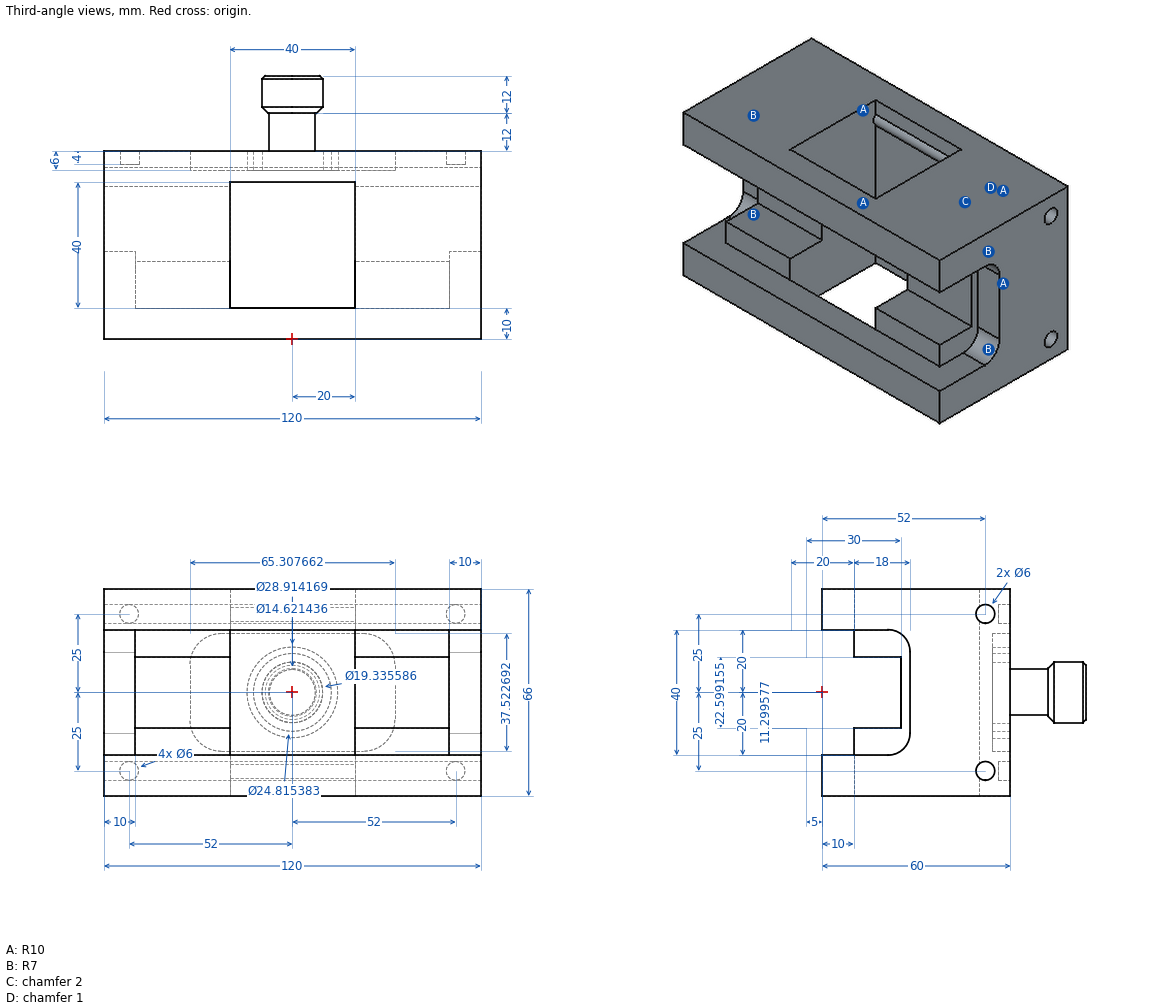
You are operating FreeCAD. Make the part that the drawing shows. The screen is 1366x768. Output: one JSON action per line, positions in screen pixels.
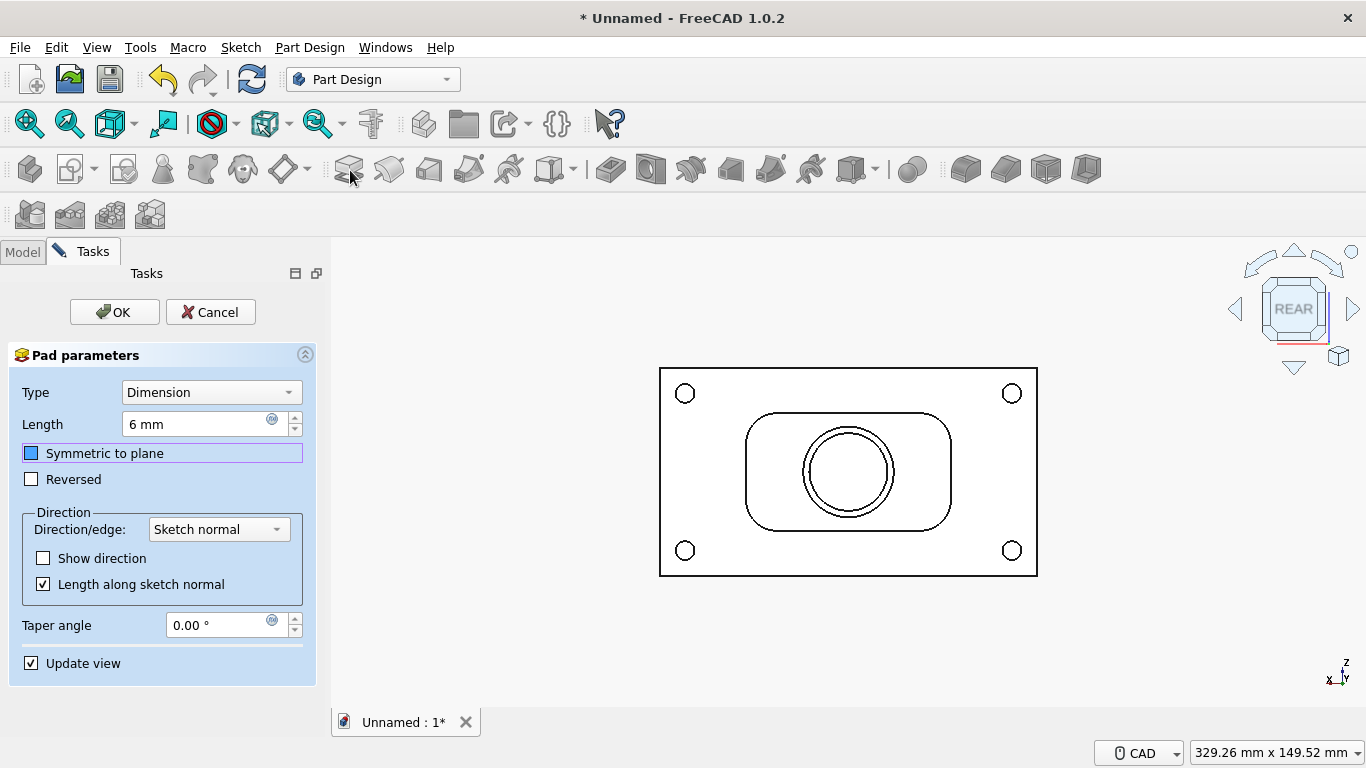
{"action": "left_click", "coordinate": [115, 312]}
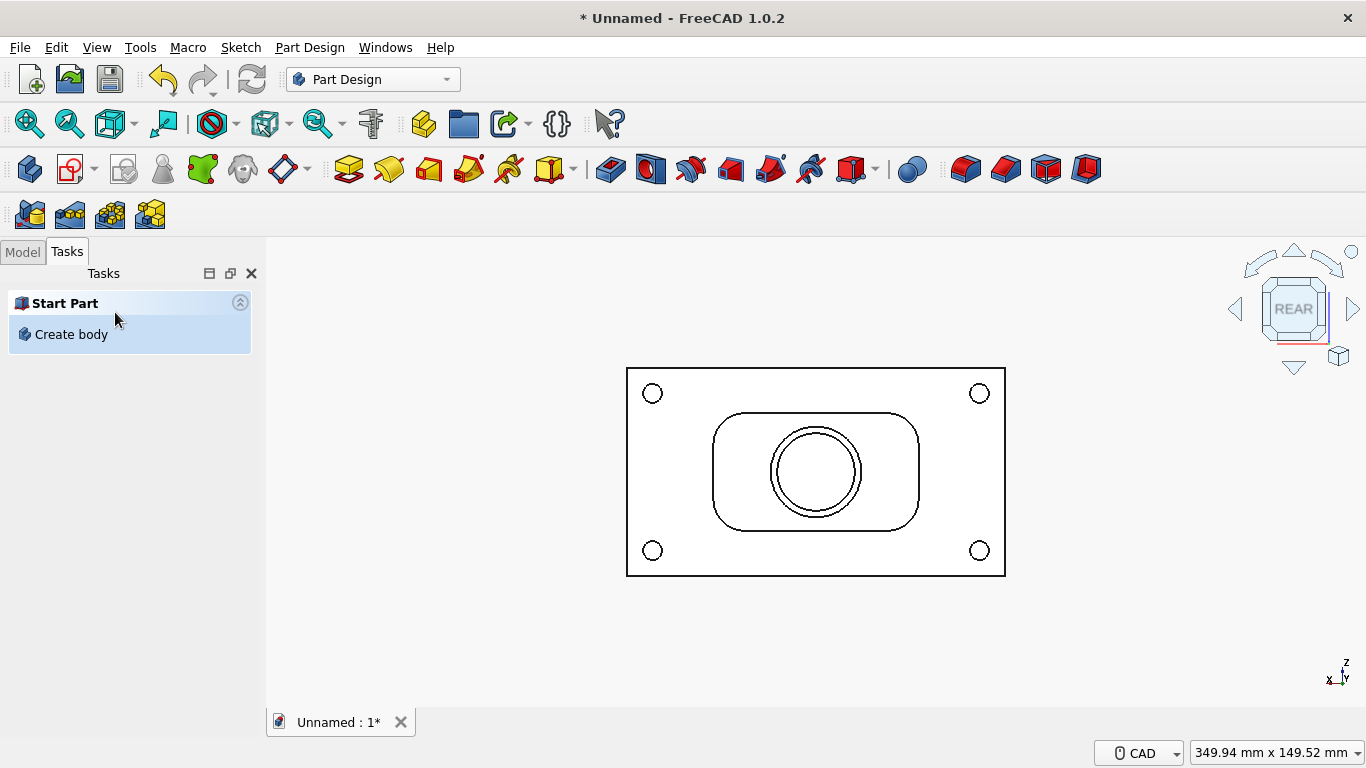
{"action": "left_click", "coordinate": [30, 124]}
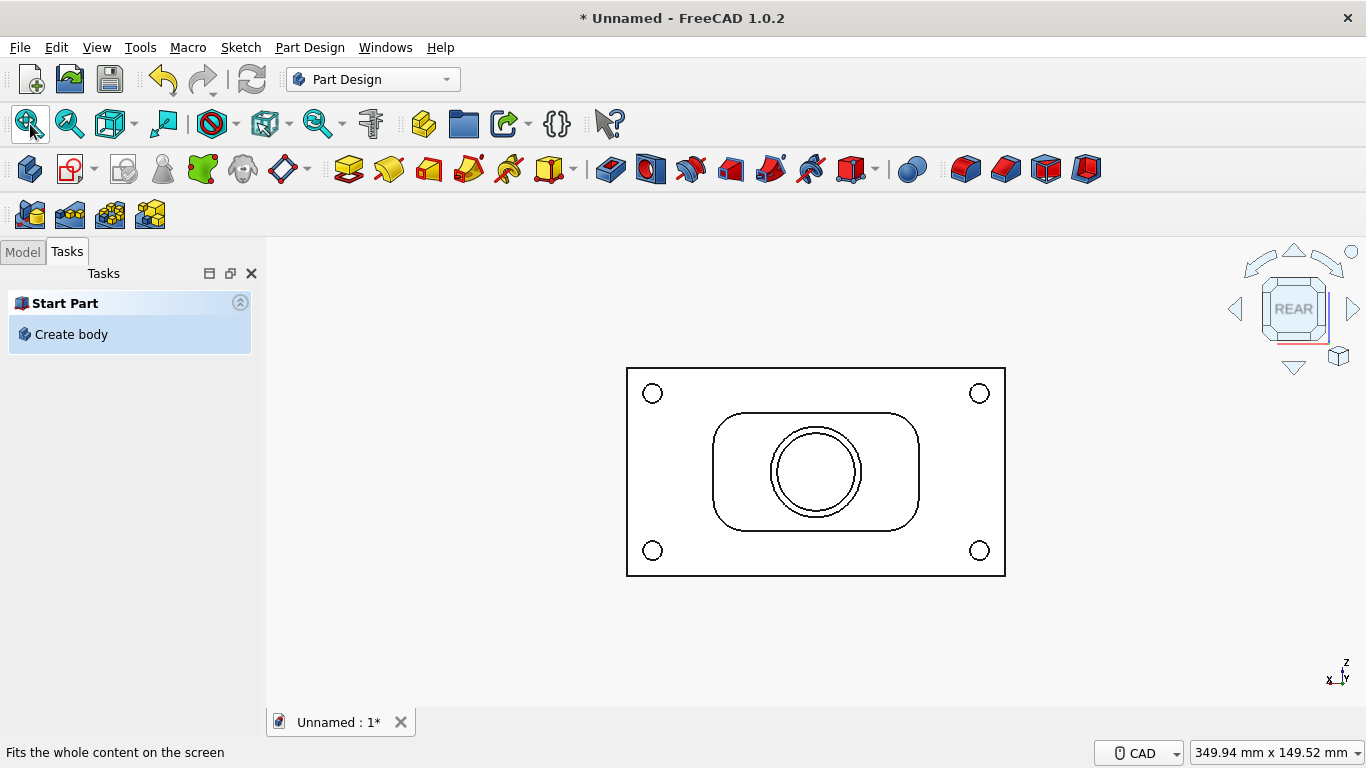
{"action": "left_click", "coordinate": [757, 505]}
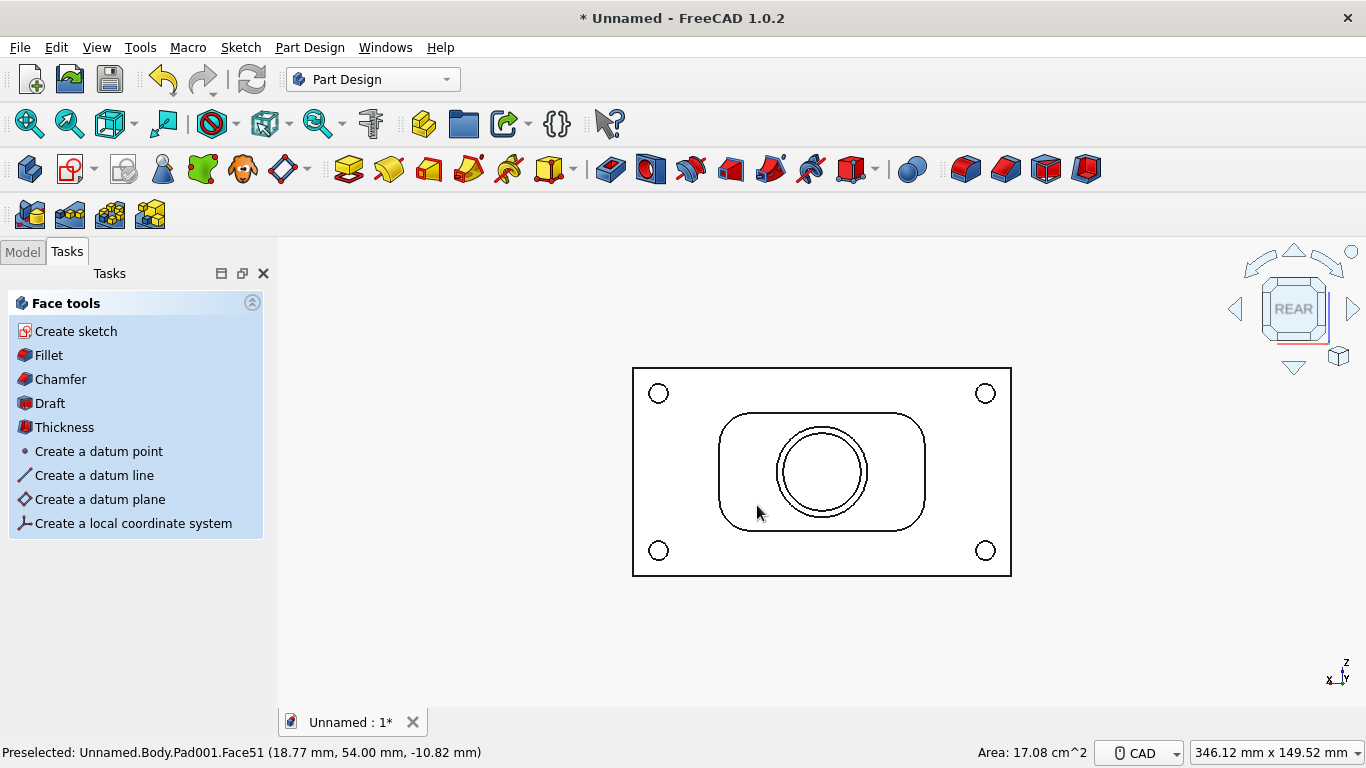
{"action": "left_click", "coordinate": [70, 170]}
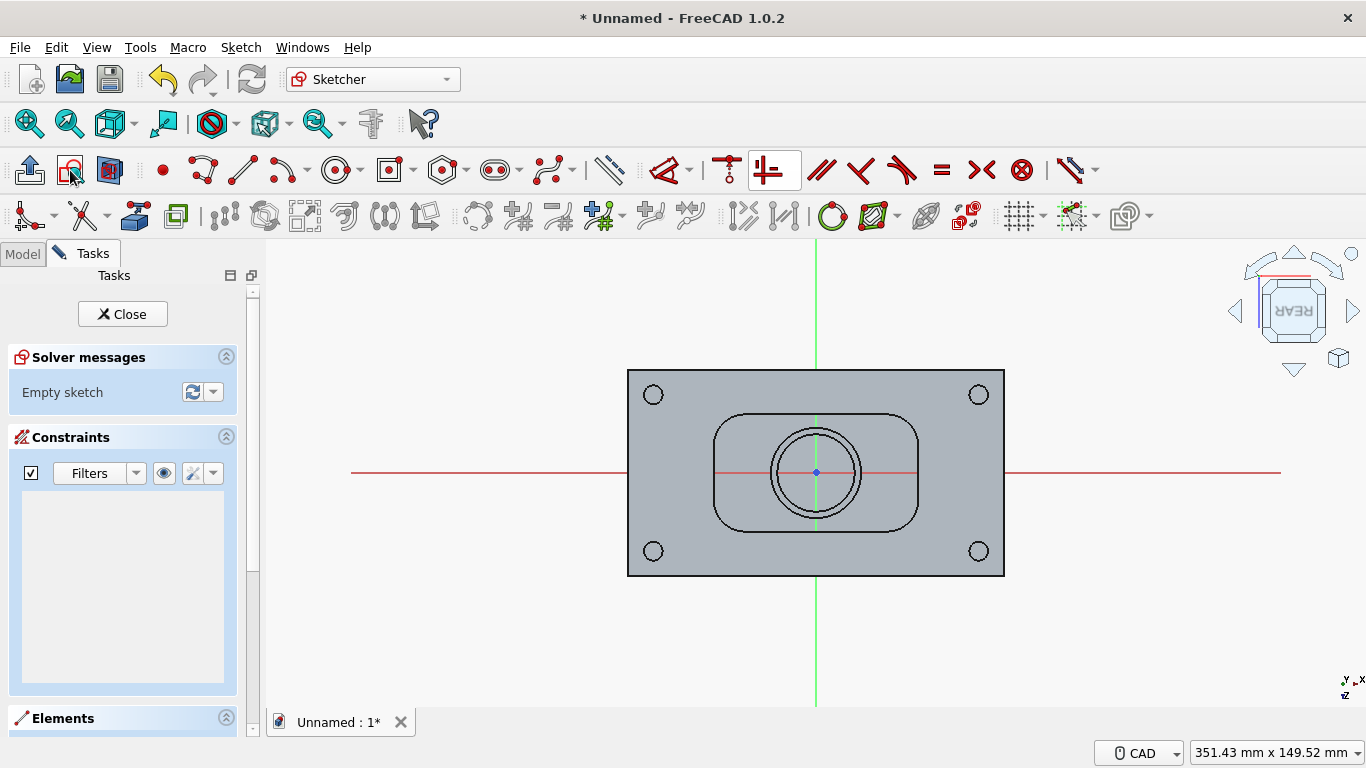
{"action": "left_click", "coordinate": [110, 170]}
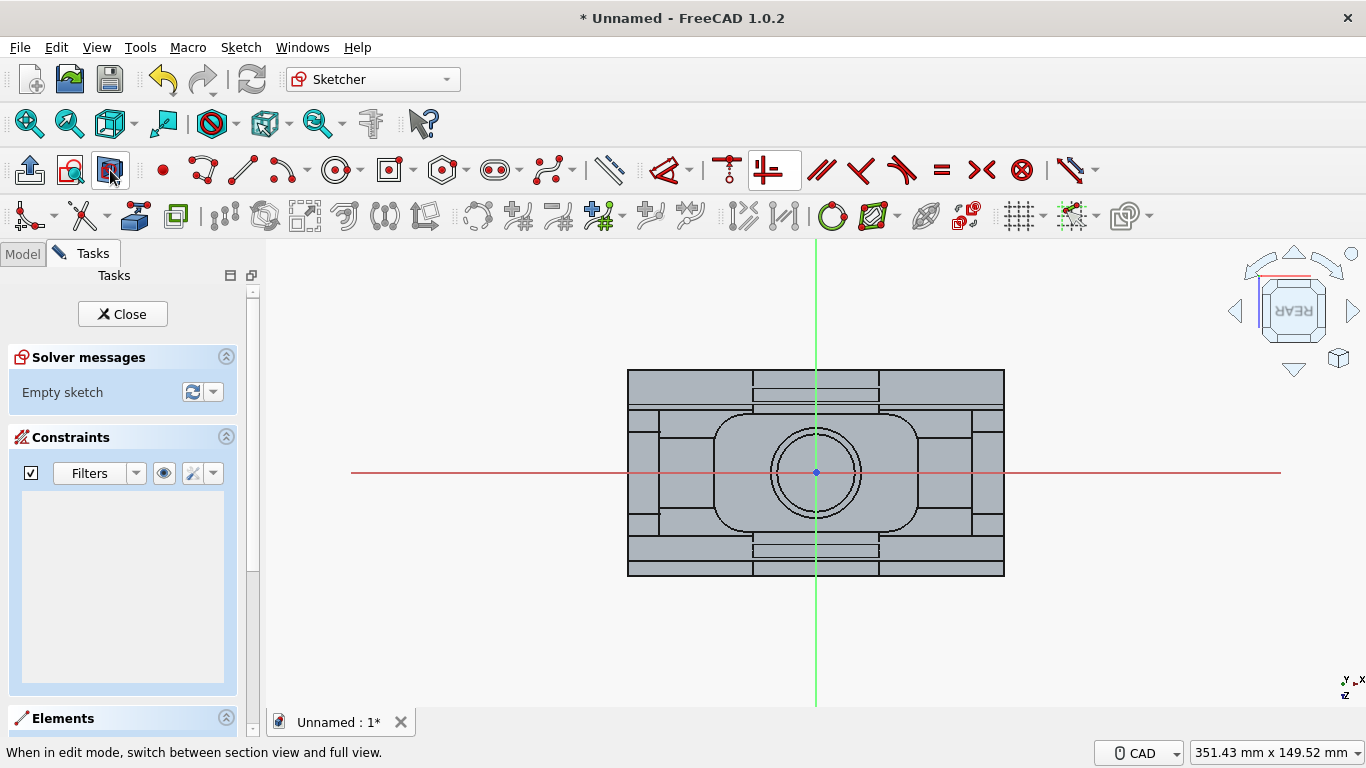
{"action": "scroll", "coordinate": [833, 473], "scroll_direction": "up", "scroll_amount": 8}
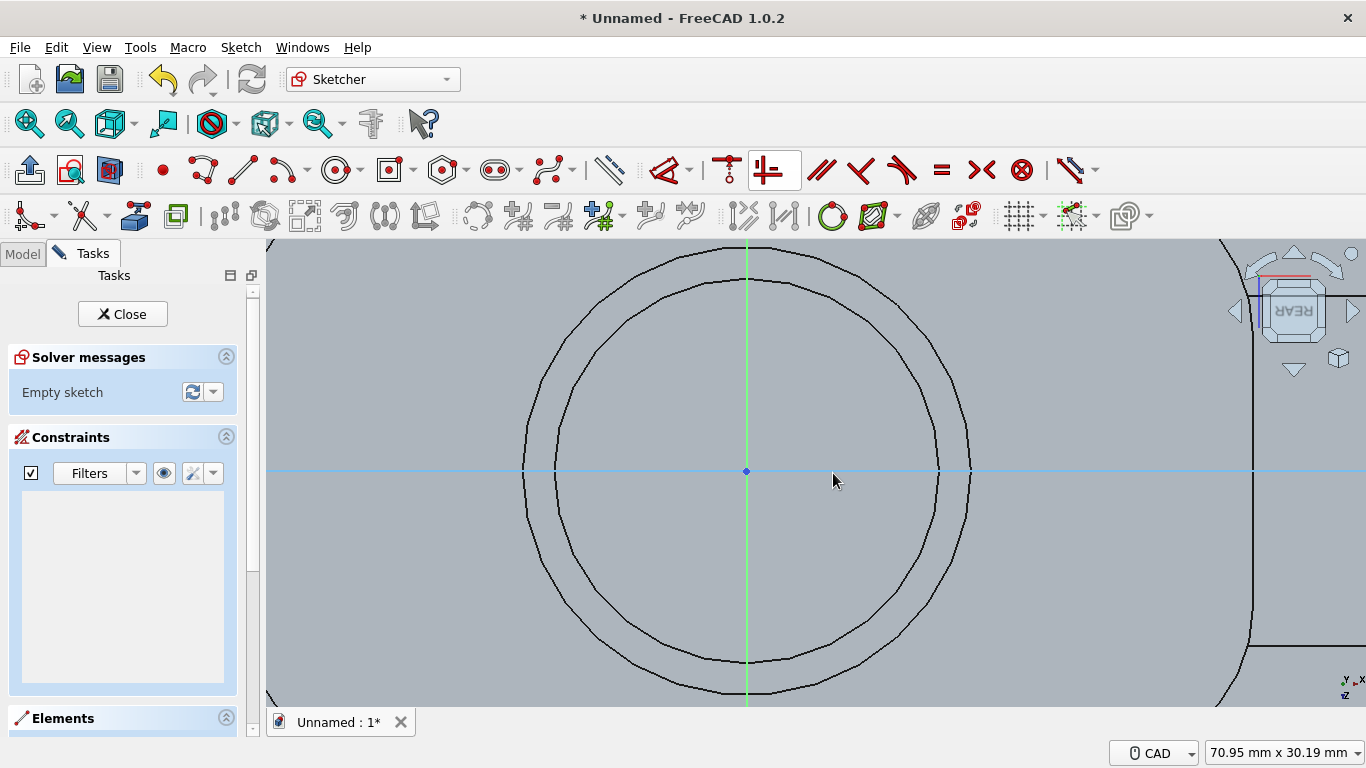
{"action": "left_click", "coordinate": [336, 170]}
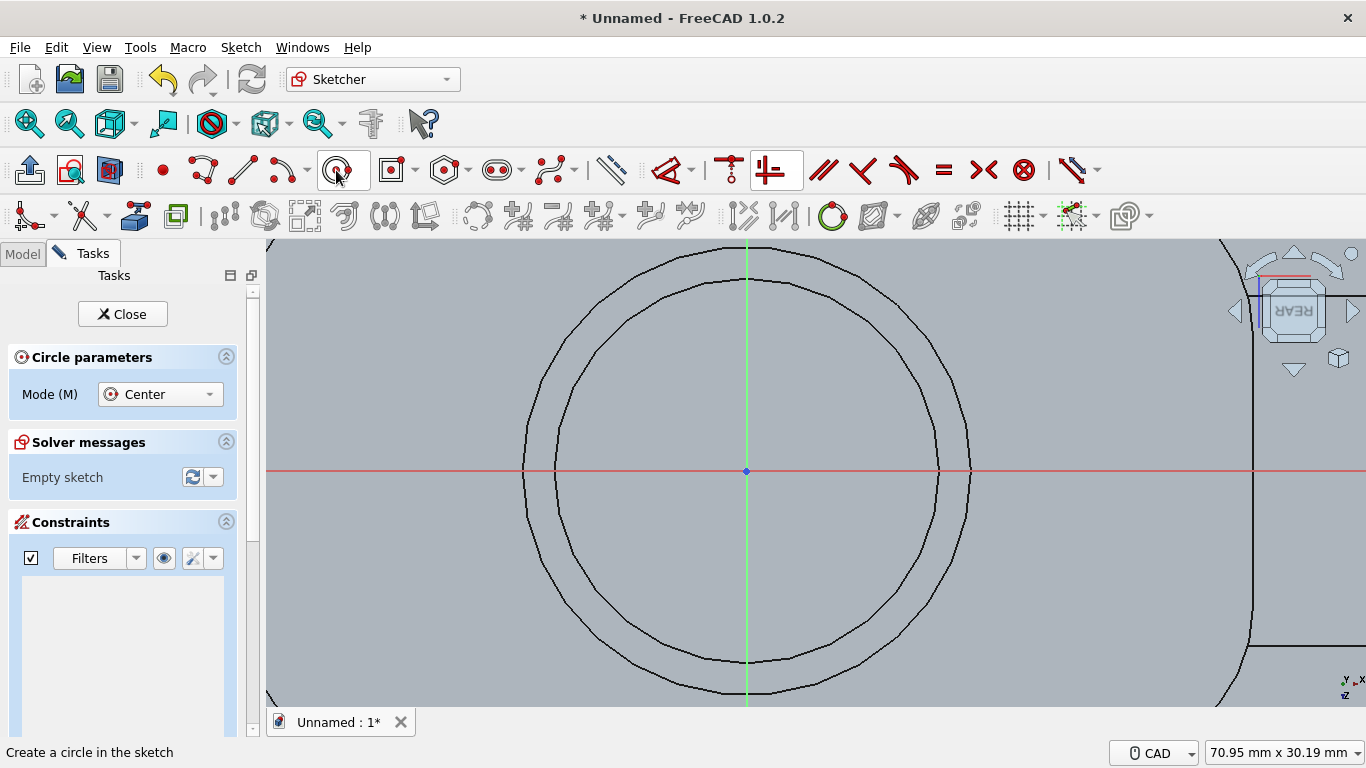
{"action": "left_click", "coordinate": [747, 471]}
{"action": "mouse_move", "coordinate": [853, 365]}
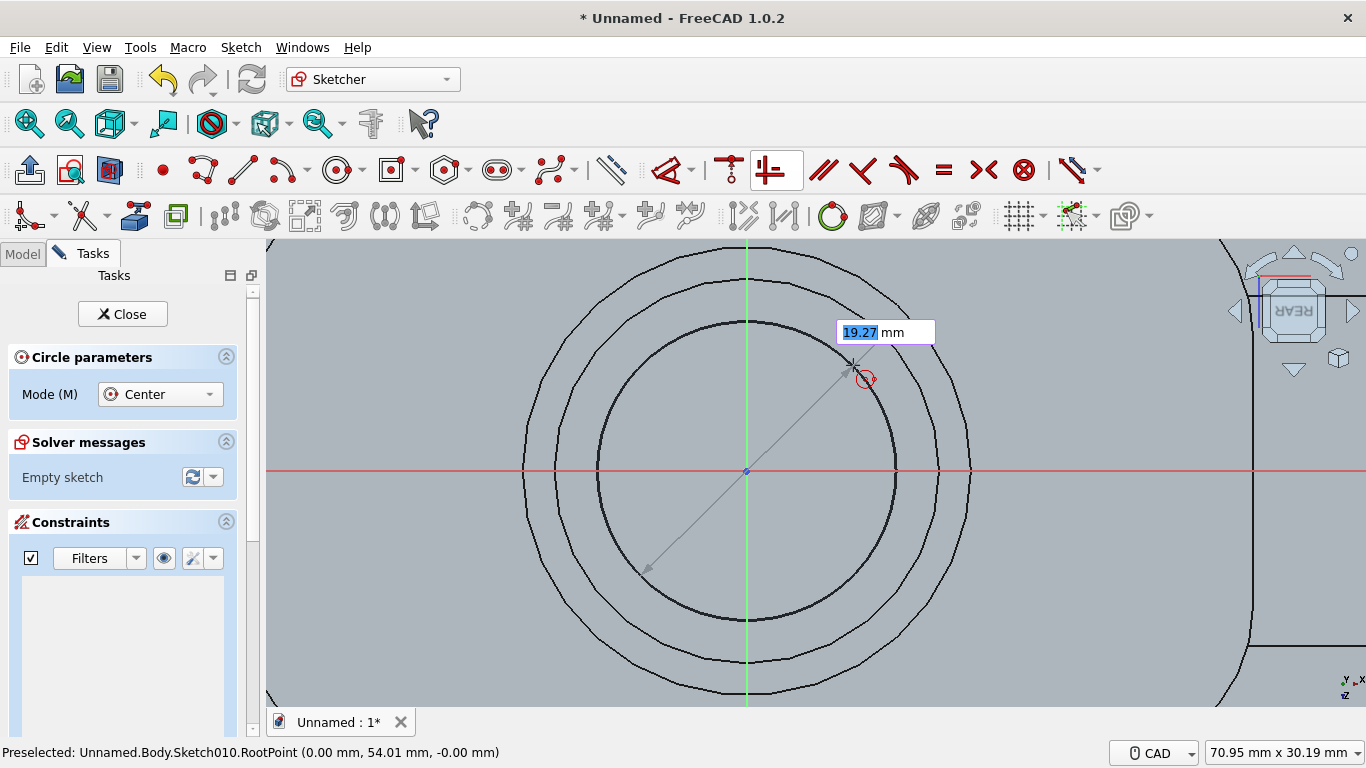
{"action": "type", "text": "19.335586"}
{"action": "key", "text": "Return"}
{"action": "key", "text": "Escape"}